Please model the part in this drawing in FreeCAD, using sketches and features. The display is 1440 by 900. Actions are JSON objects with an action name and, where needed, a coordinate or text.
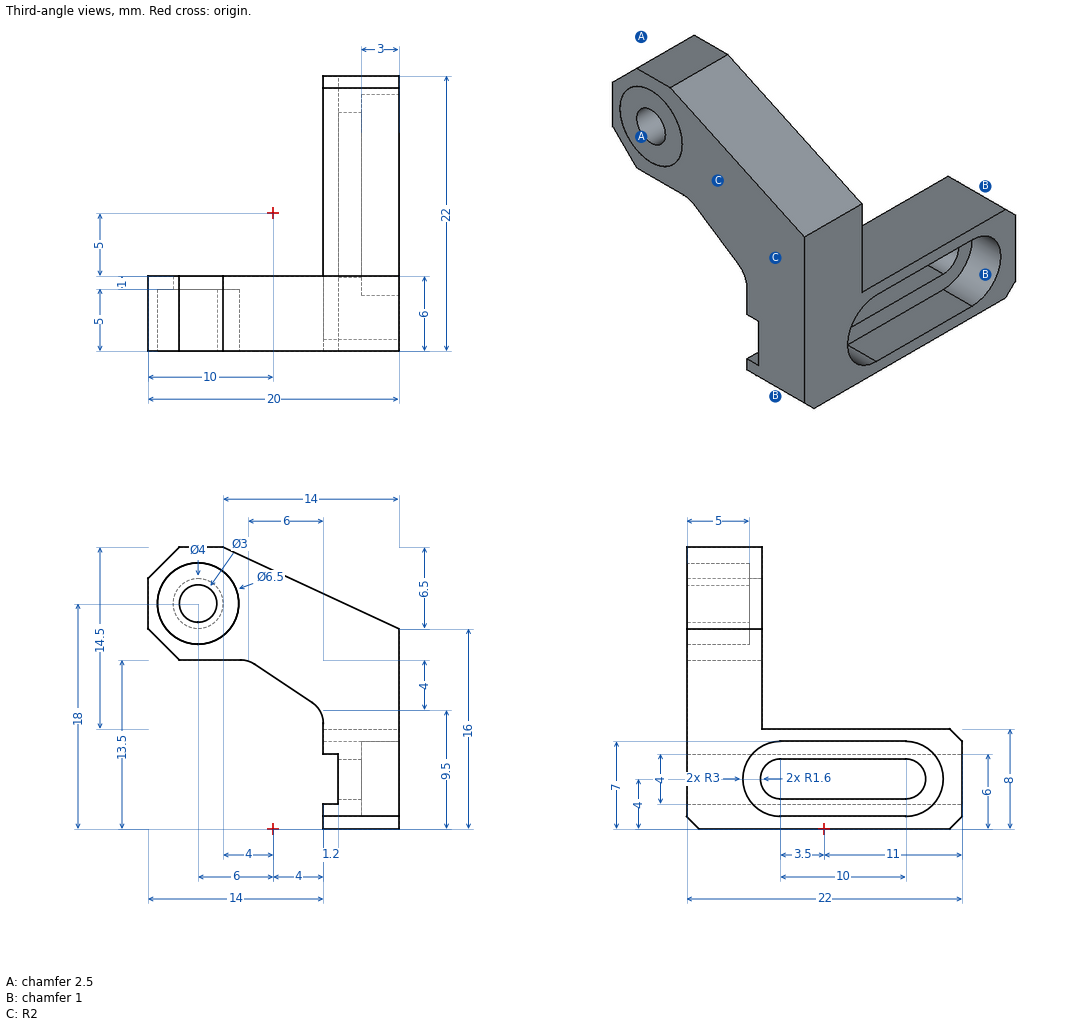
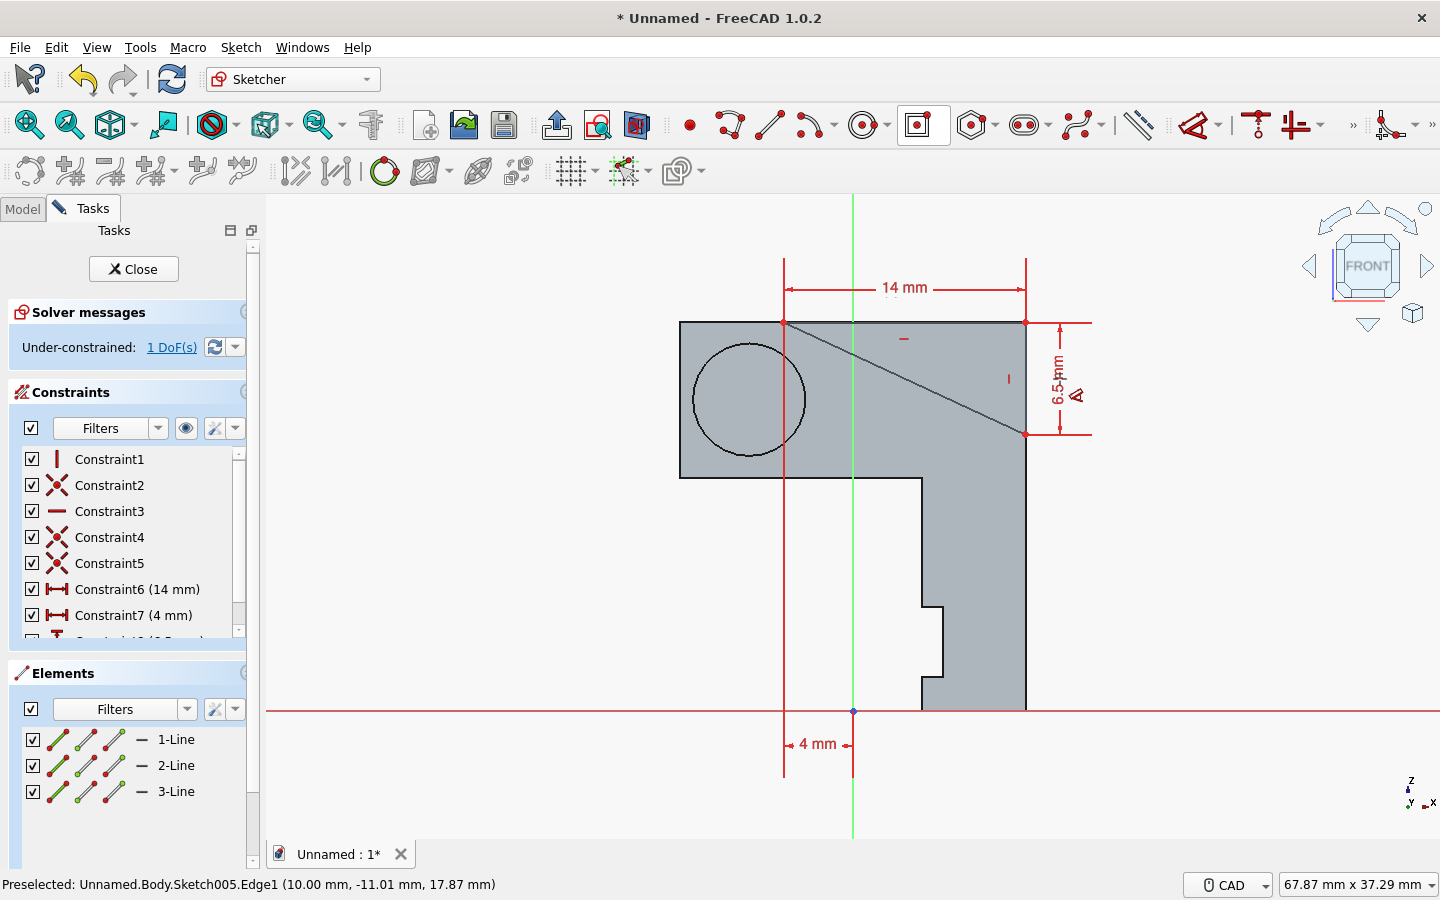
{"action": "left_click", "coordinate": [1026, 435]}
{"action": "left_click", "coordinate": [1060, 573]}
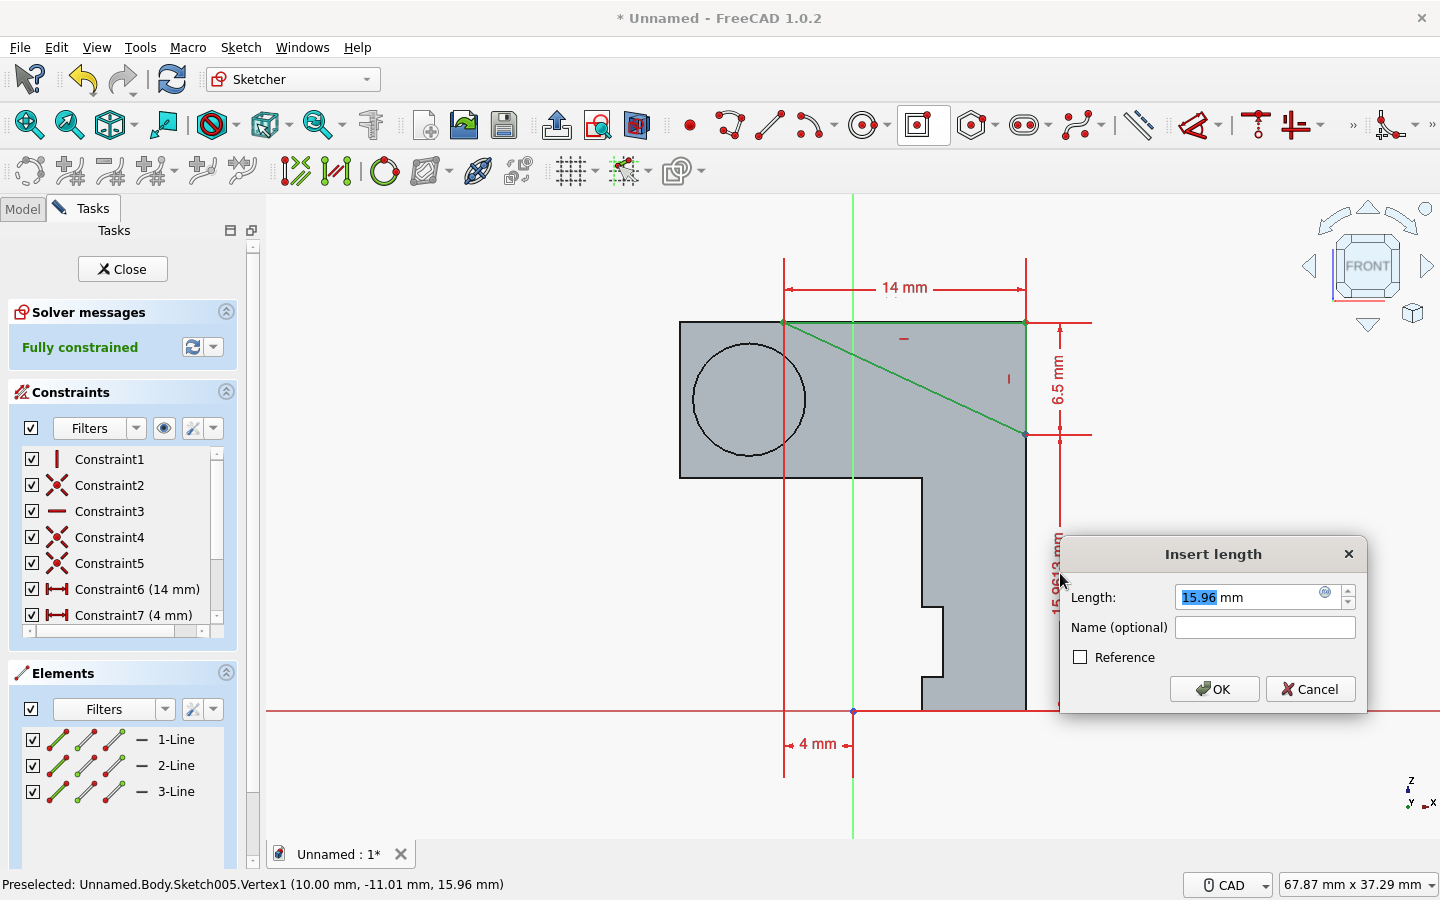
{"action": "type", "text": "16"}
{"action": "key", "text": "Return"}
{"action": "key", "text": "Escape"}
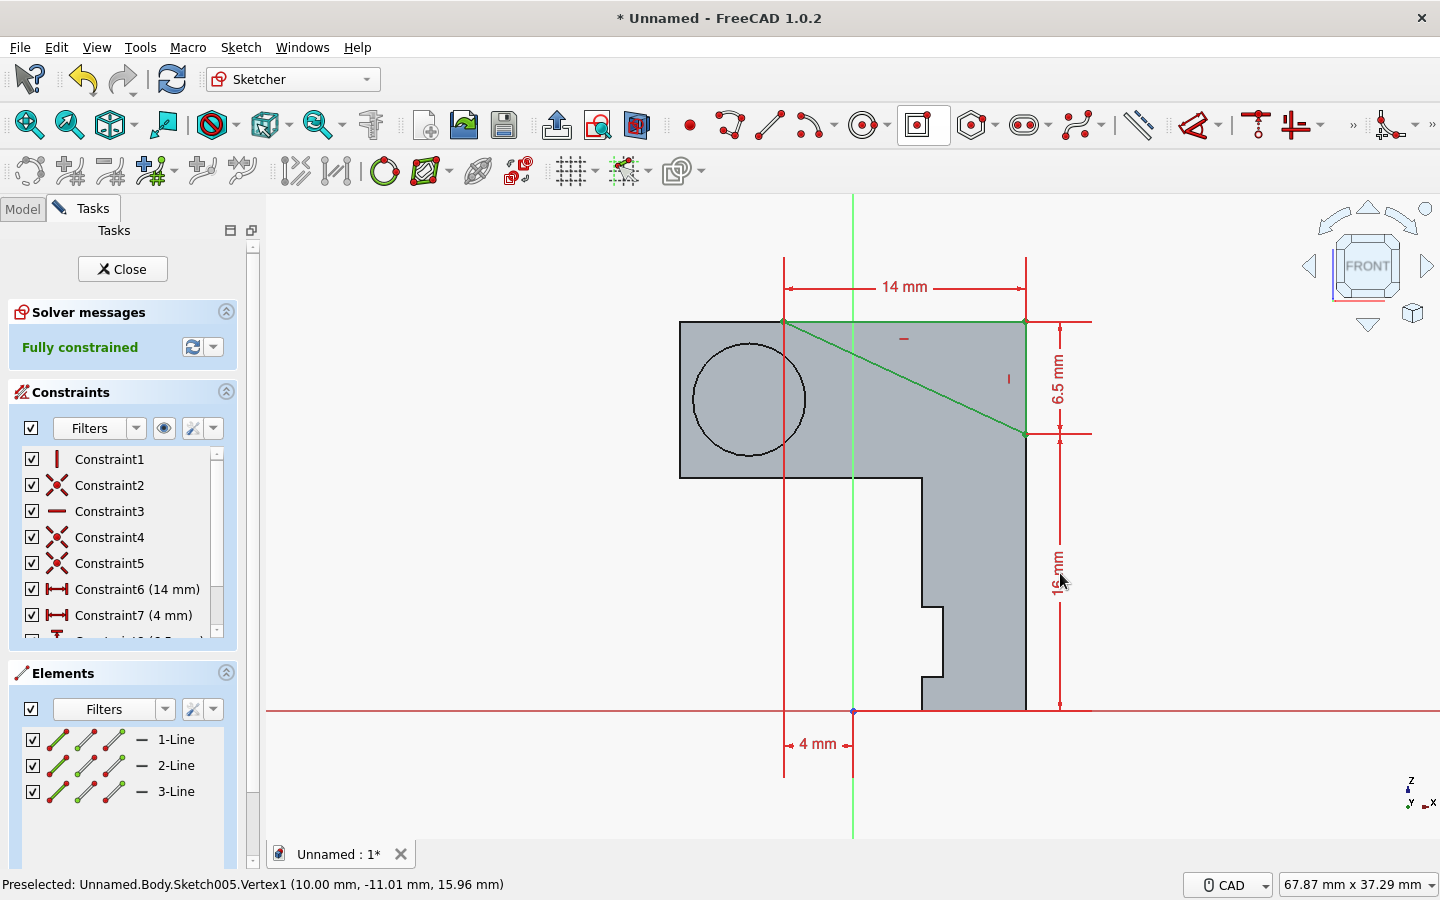
{"action": "left_click", "coordinate": [123, 269]}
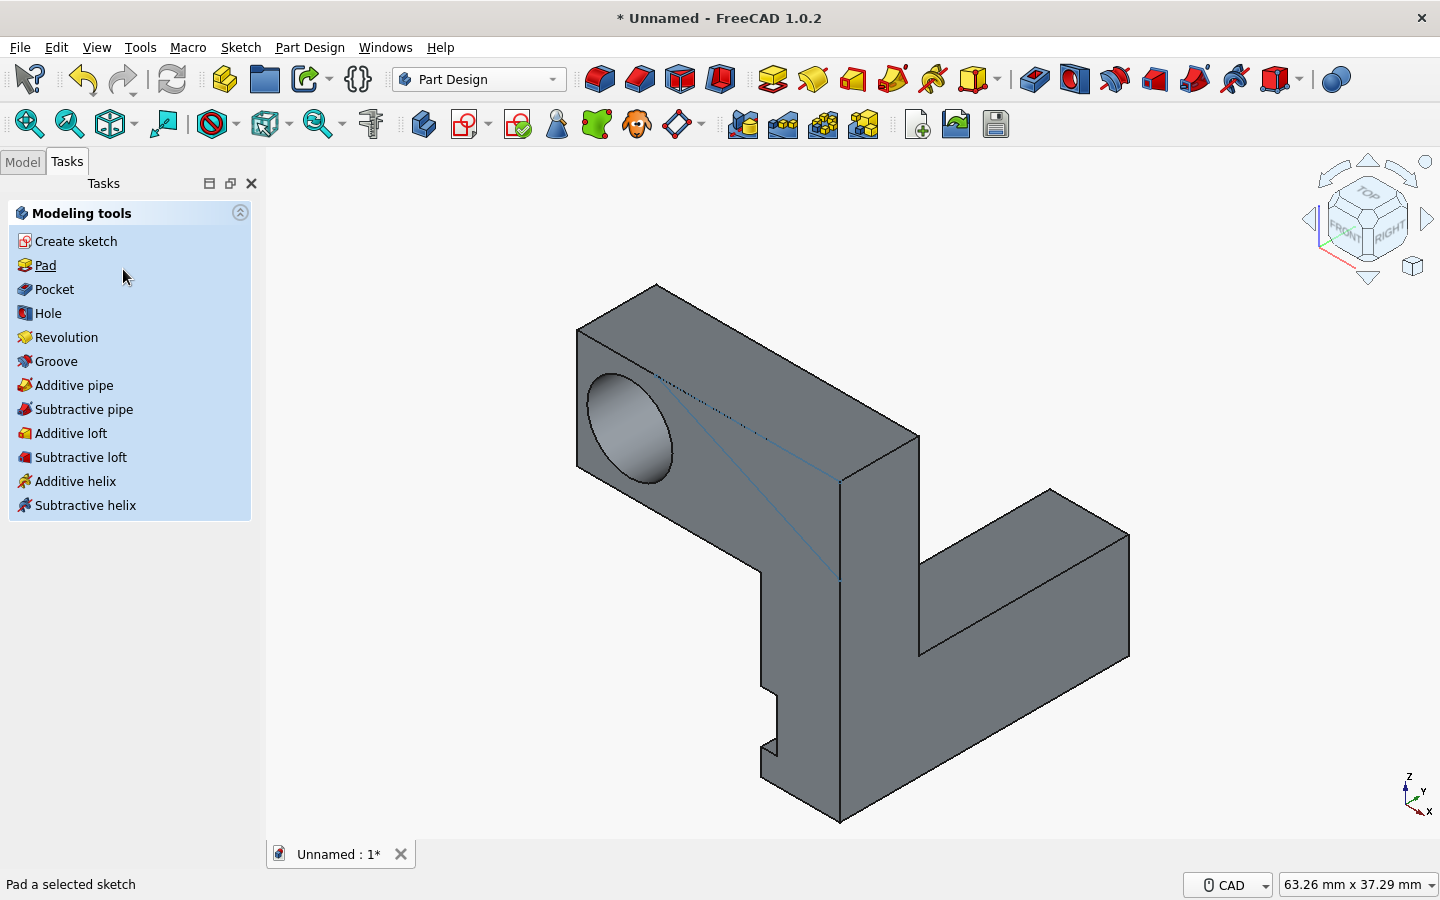
{"action": "left_click", "coordinate": [1036, 80]}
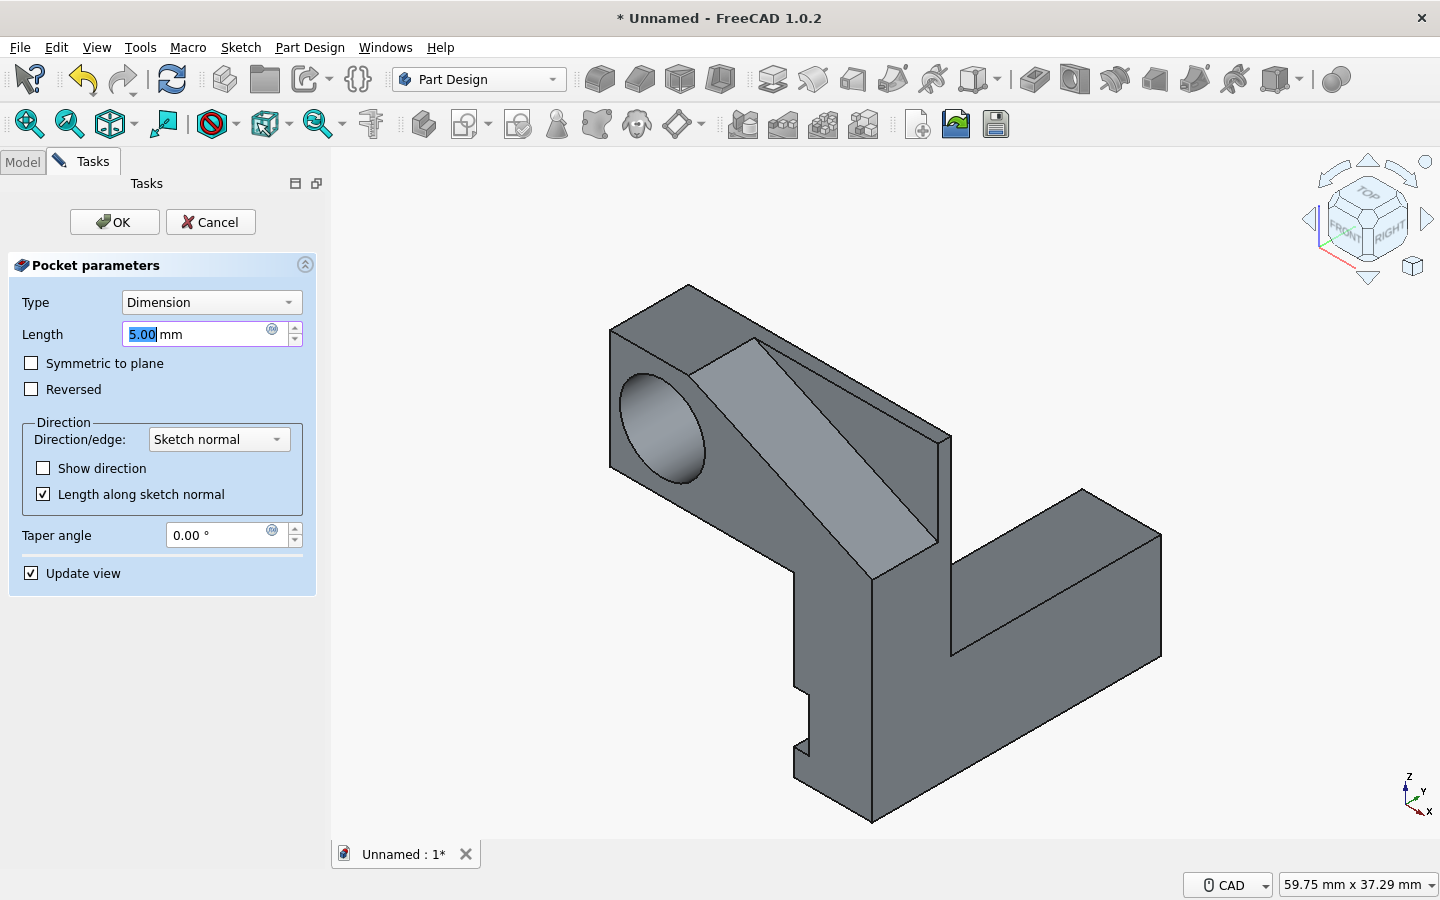
{"action": "left_click", "coordinate": [212, 302]}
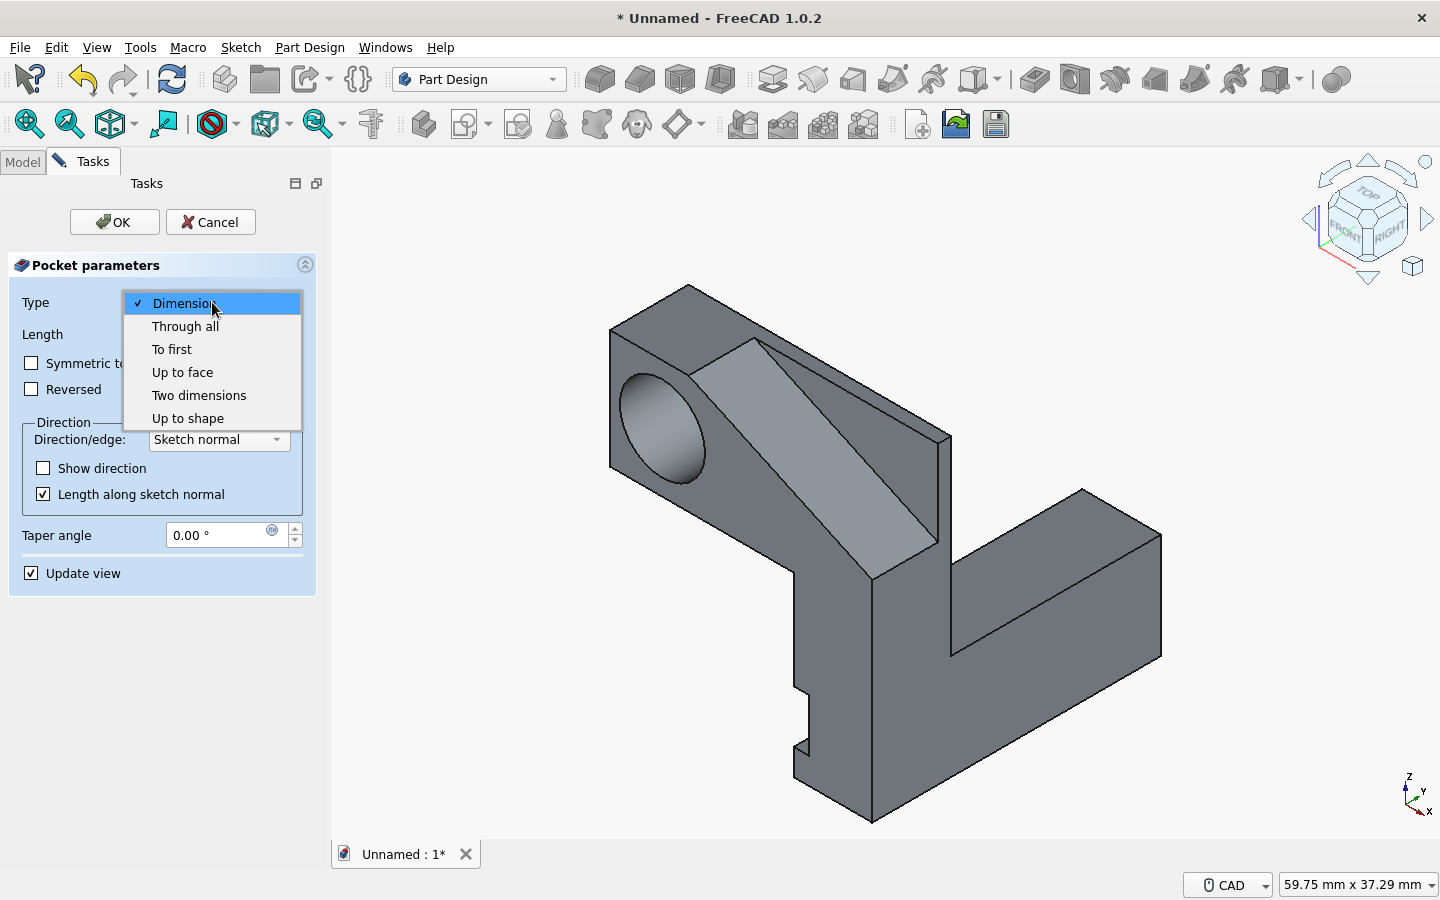
{"action": "left_click", "coordinate": [212, 326]}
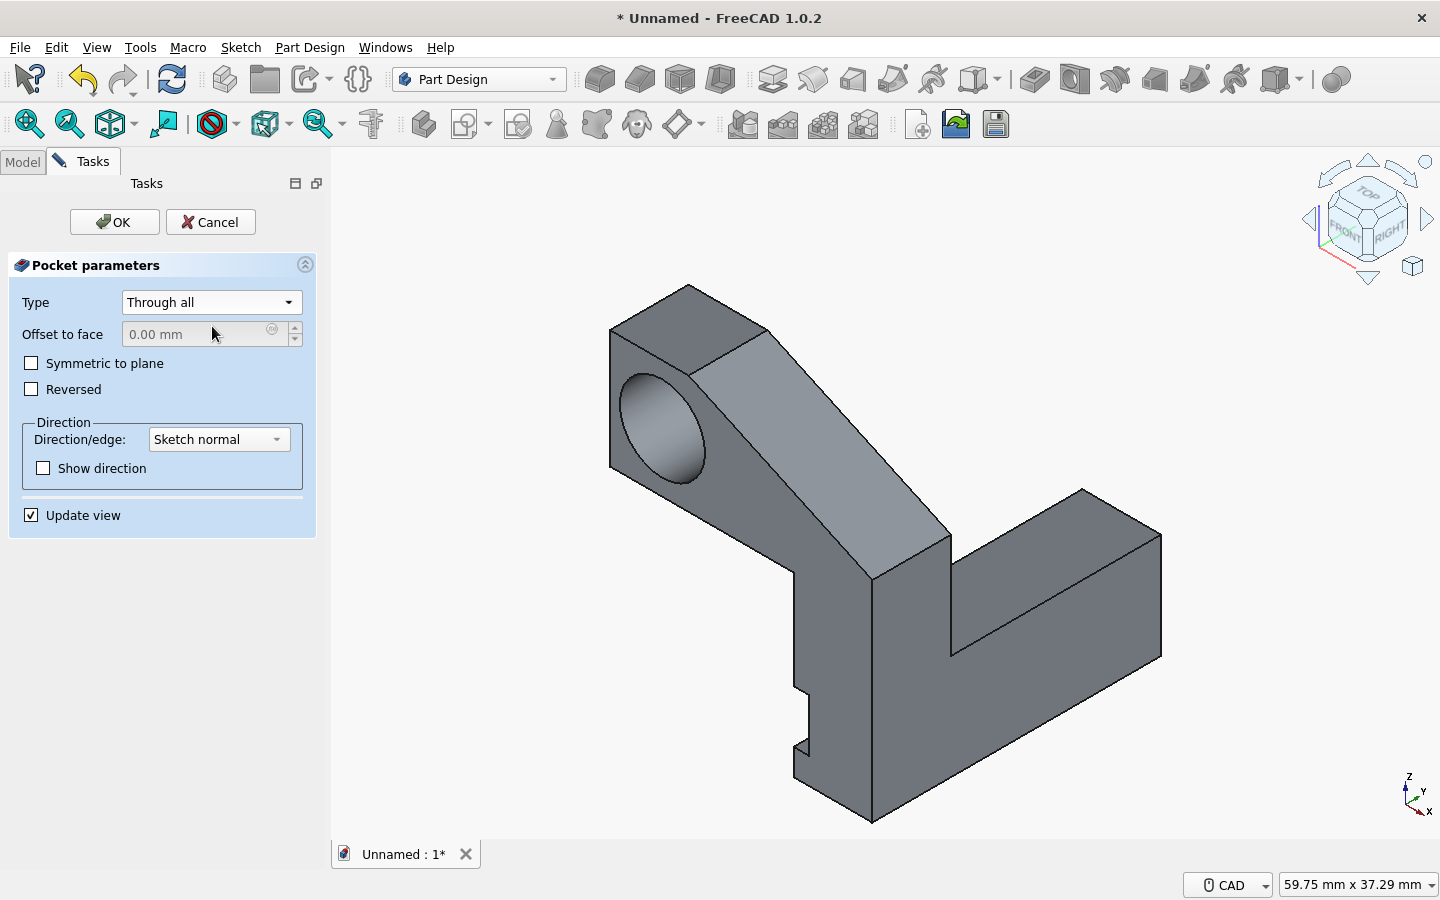
{"action": "left_click", "coordinate": [115, 222]}